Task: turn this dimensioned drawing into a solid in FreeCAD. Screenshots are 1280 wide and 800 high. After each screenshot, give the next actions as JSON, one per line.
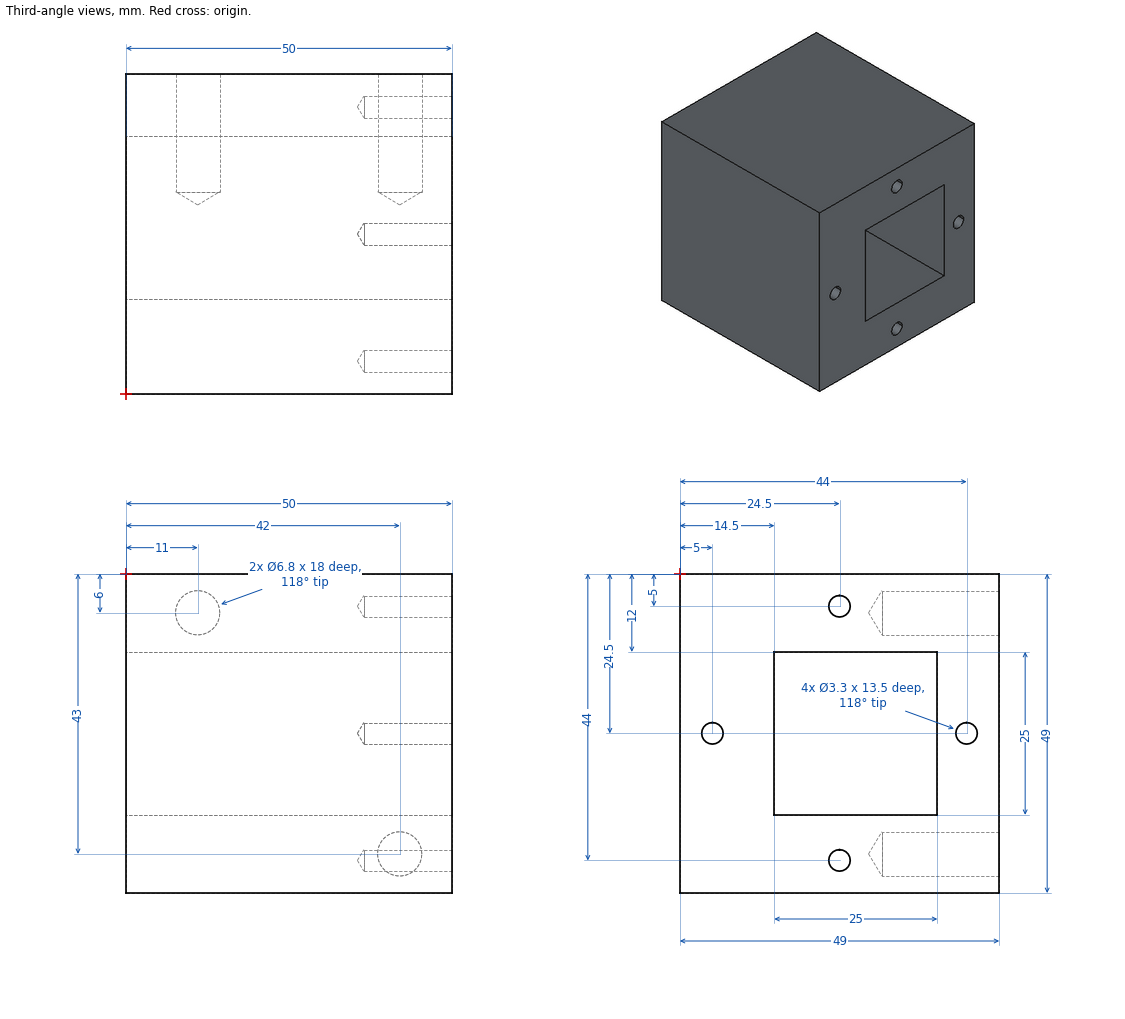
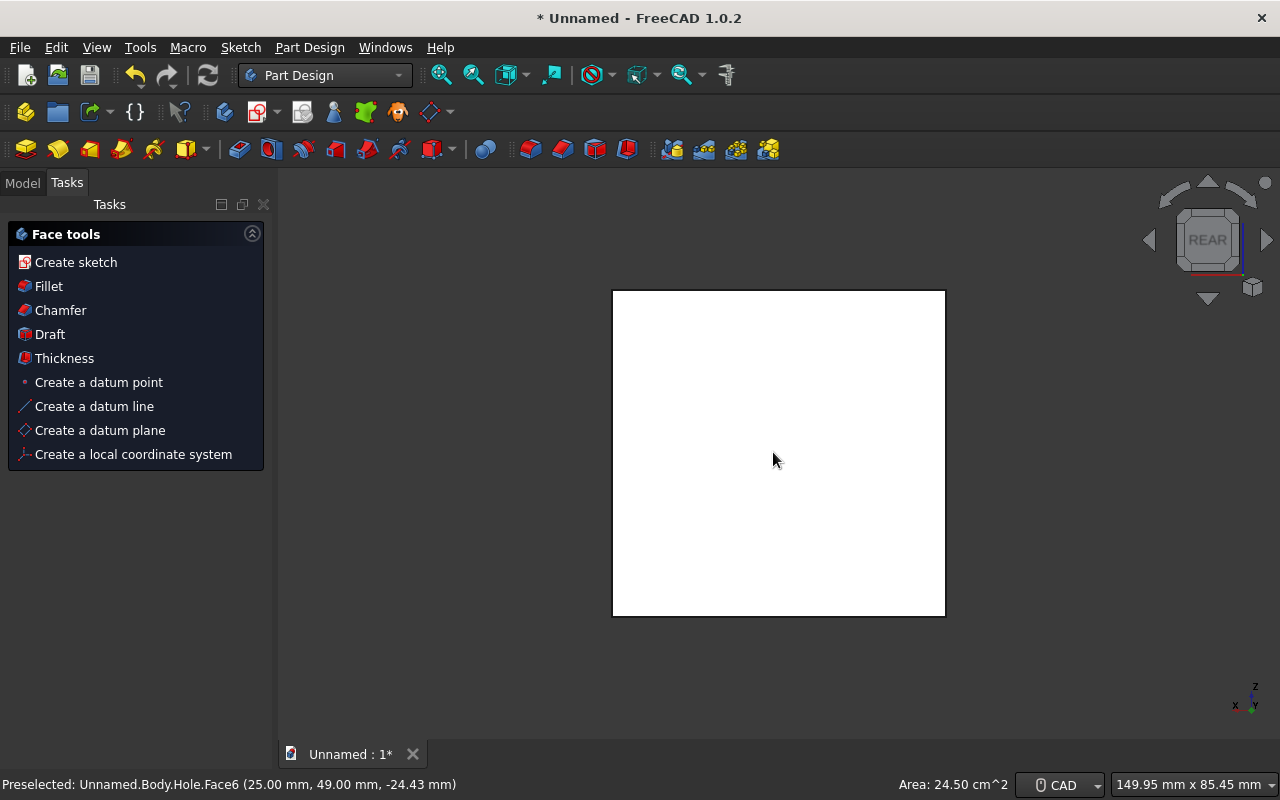
{"action": "left_click", "coordinate": [258, 112]}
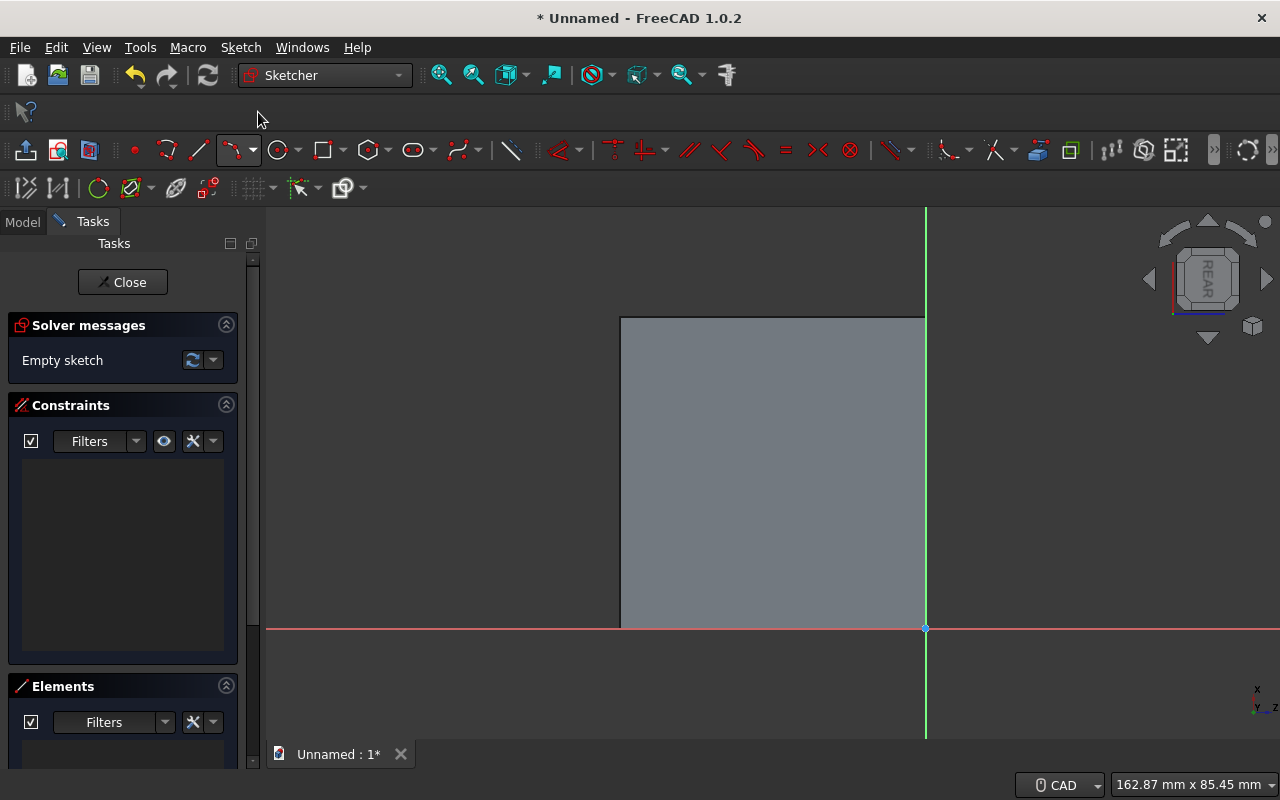
{"action": "key", "text": "g c"}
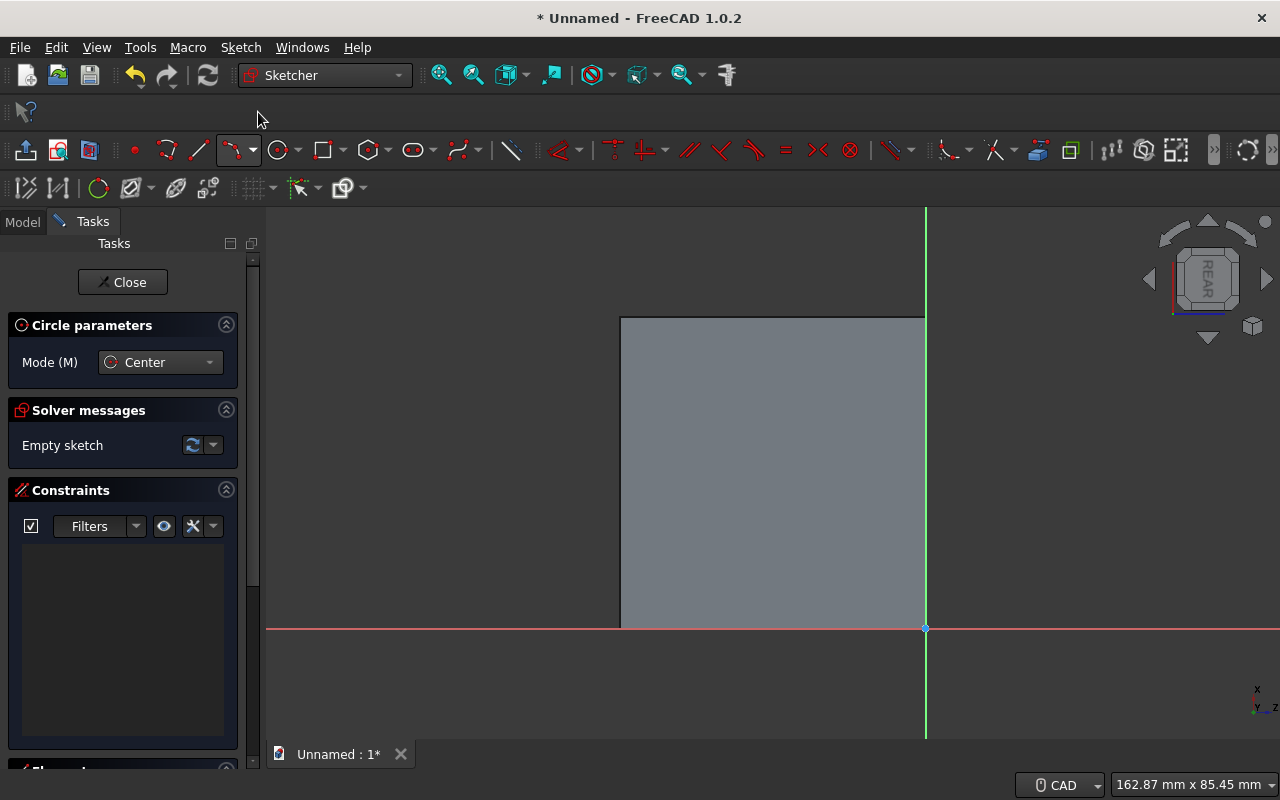
{"action": "left_click", "coordinate": [888, 560]}
{"action": "mouse_move", "coordinate": [903, 545]}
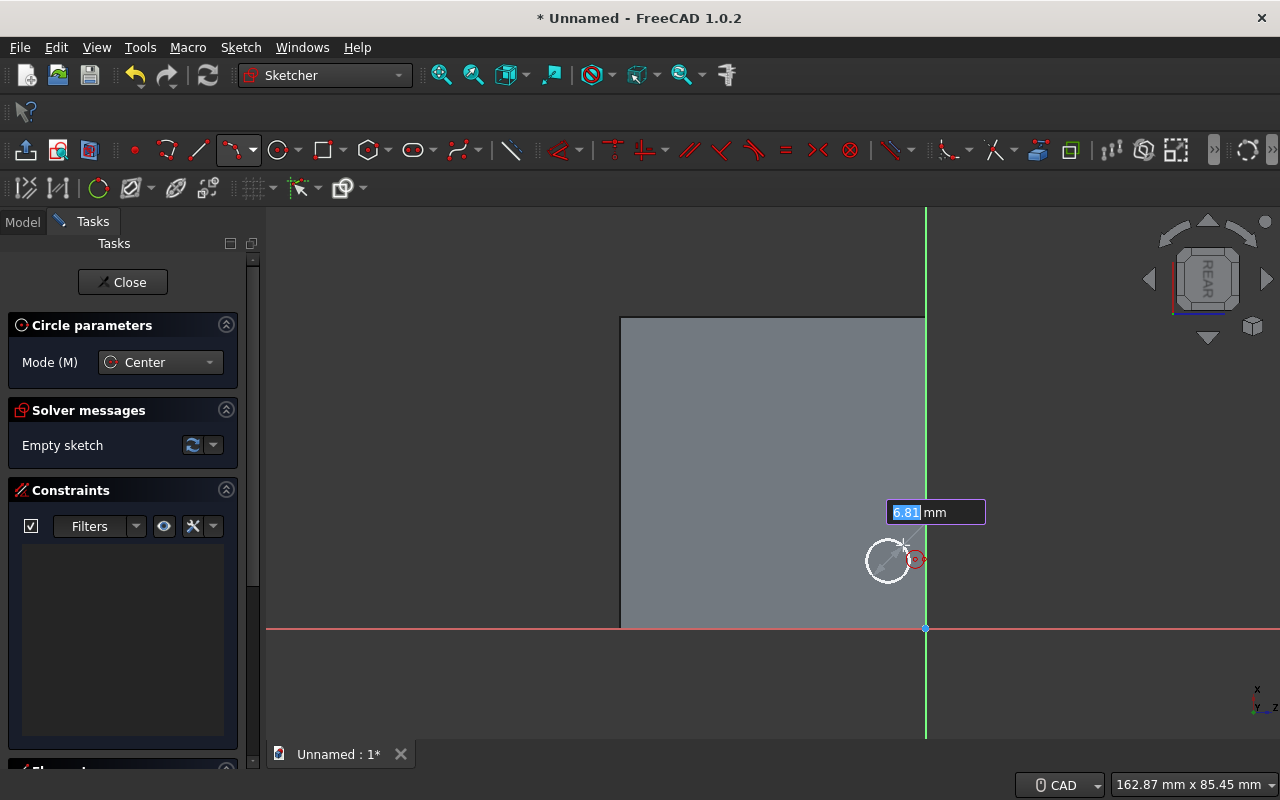
{"action": "type", "text": "6.8"}
{"action": "key", "text": "Return"}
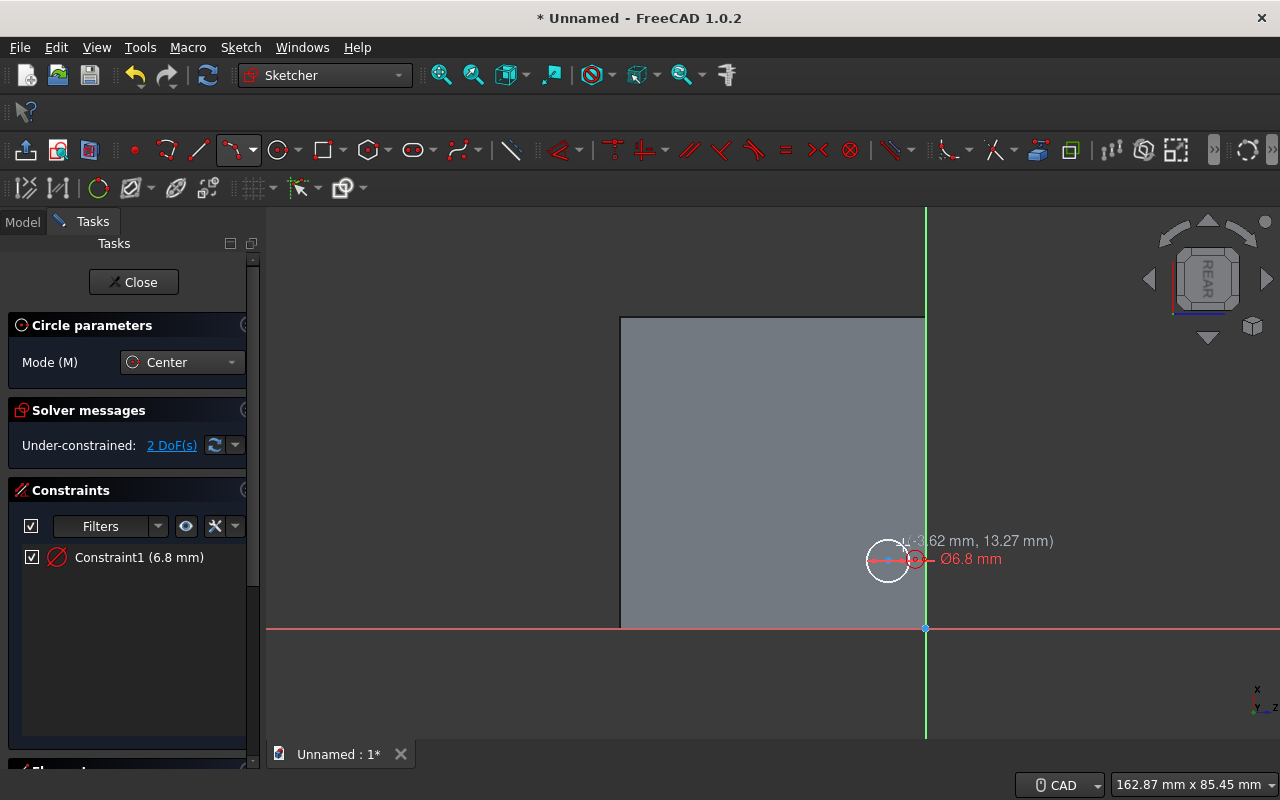
{"action": "left_click", "coordinate": [658, 367]}
{"action": "mouse_move", "coordinate": [673, 352]}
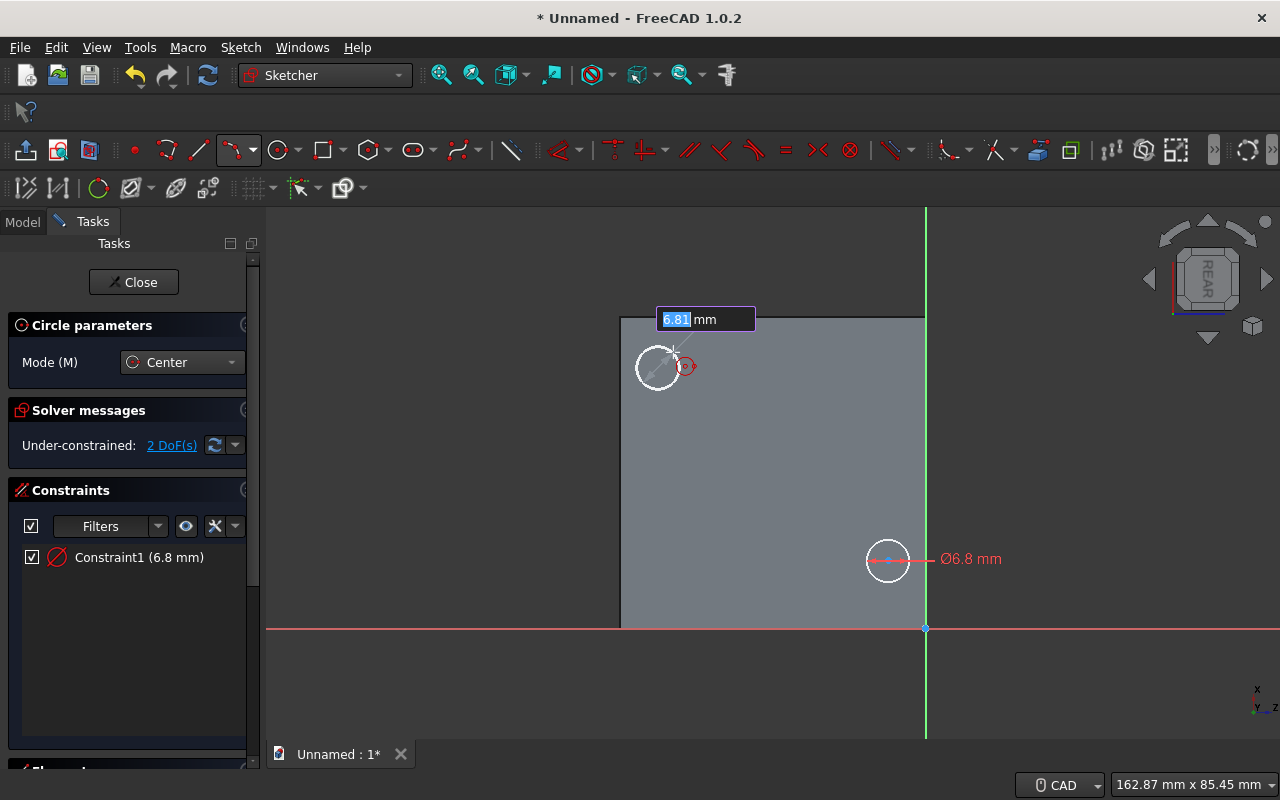
{"action": "type", "text": "6.8"}
{"action": "key", "text": "Return"}
{"action": "key", "text": "Escape"}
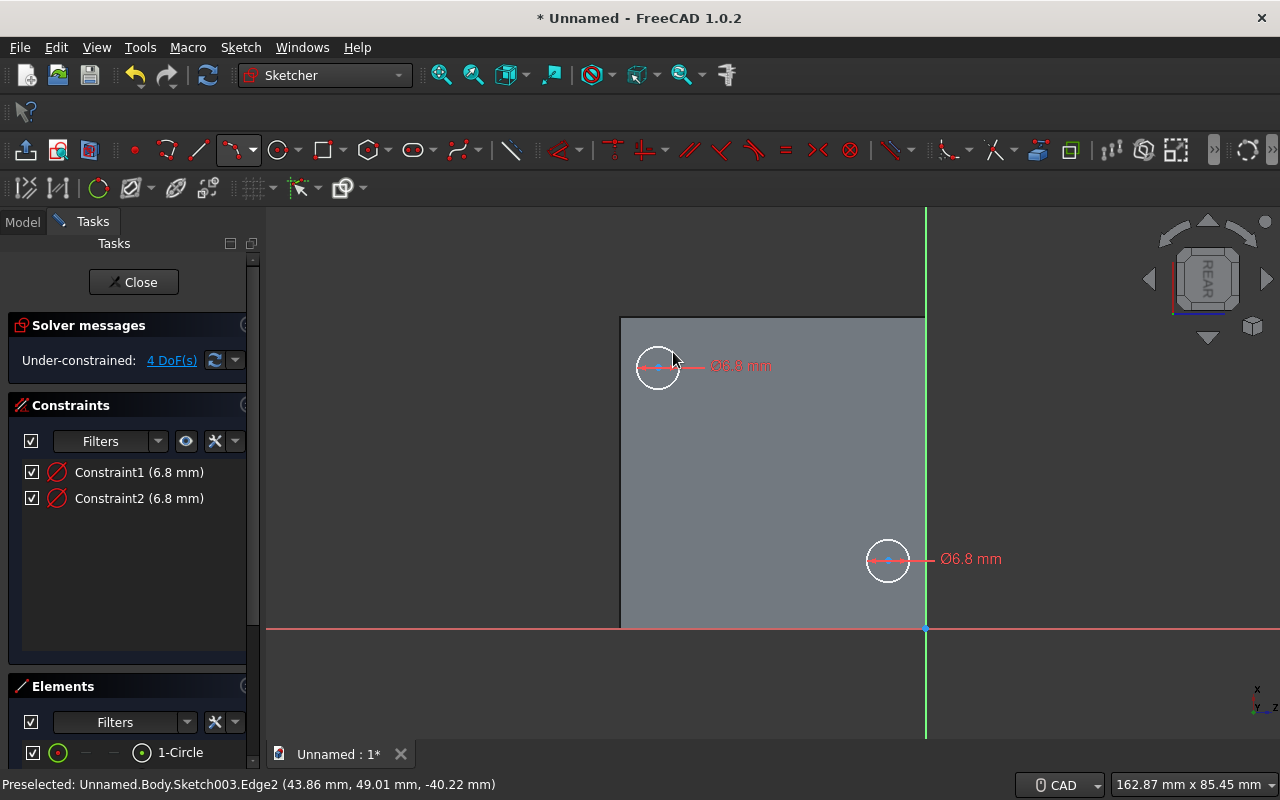
{"action": "key", "text": "d"}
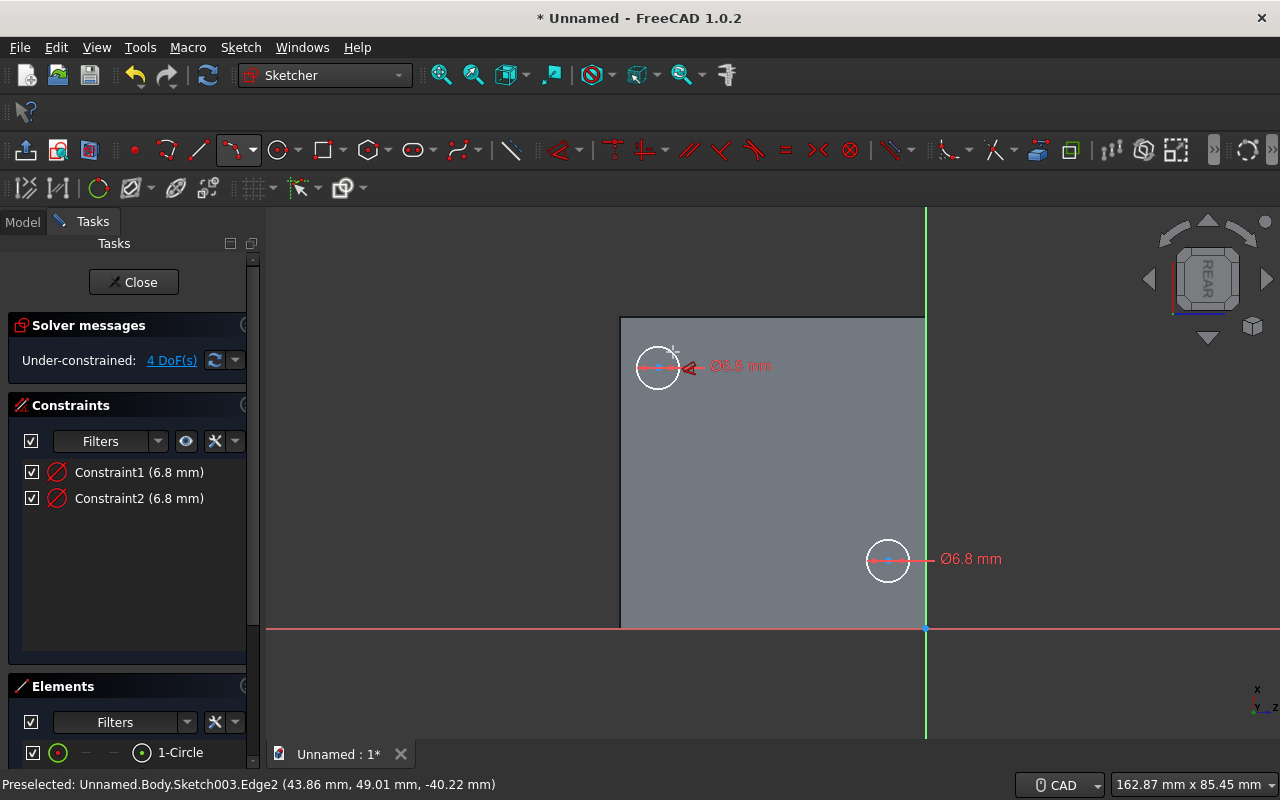
{"action": "left_click", "coordinate": [888, 561]}
{"action": "left_click", "coordinate": [907, 663]}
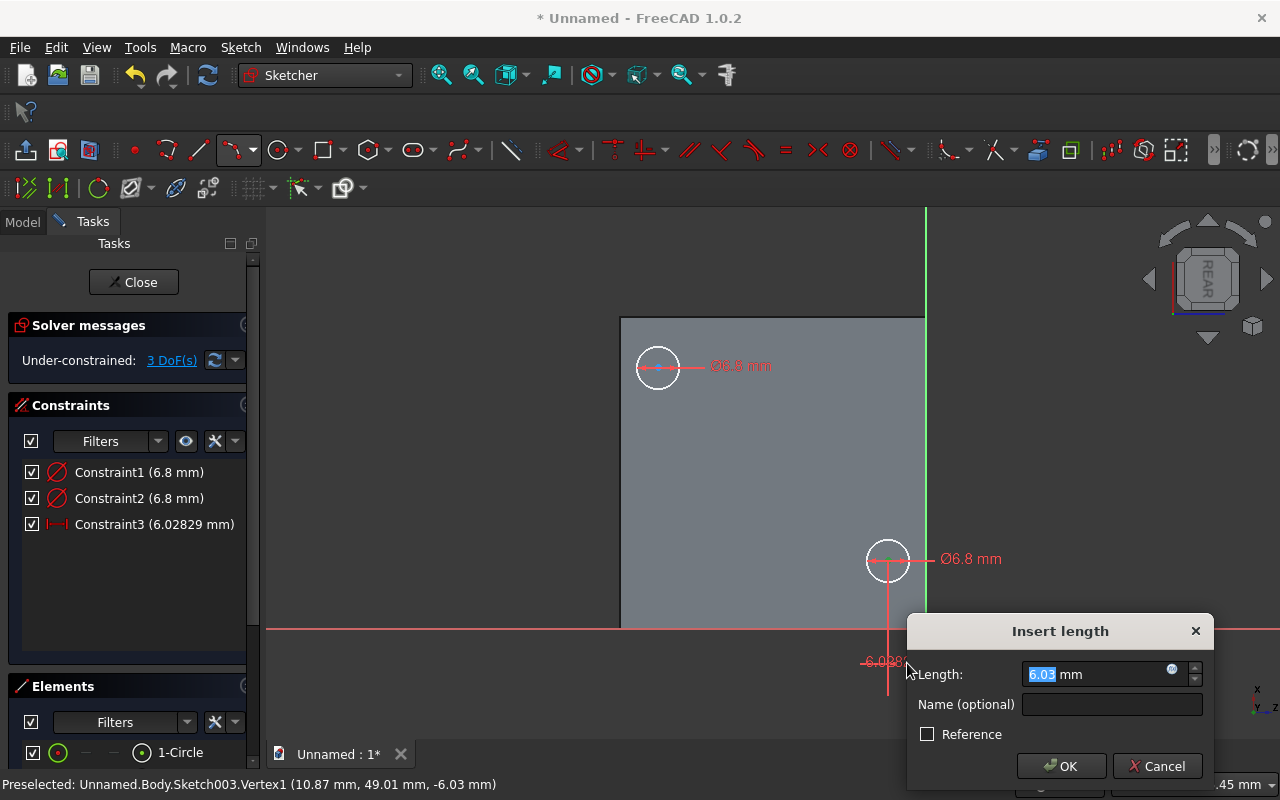
{"action": "type", "text": "6"}
{"action": "key", "text": "Return"}